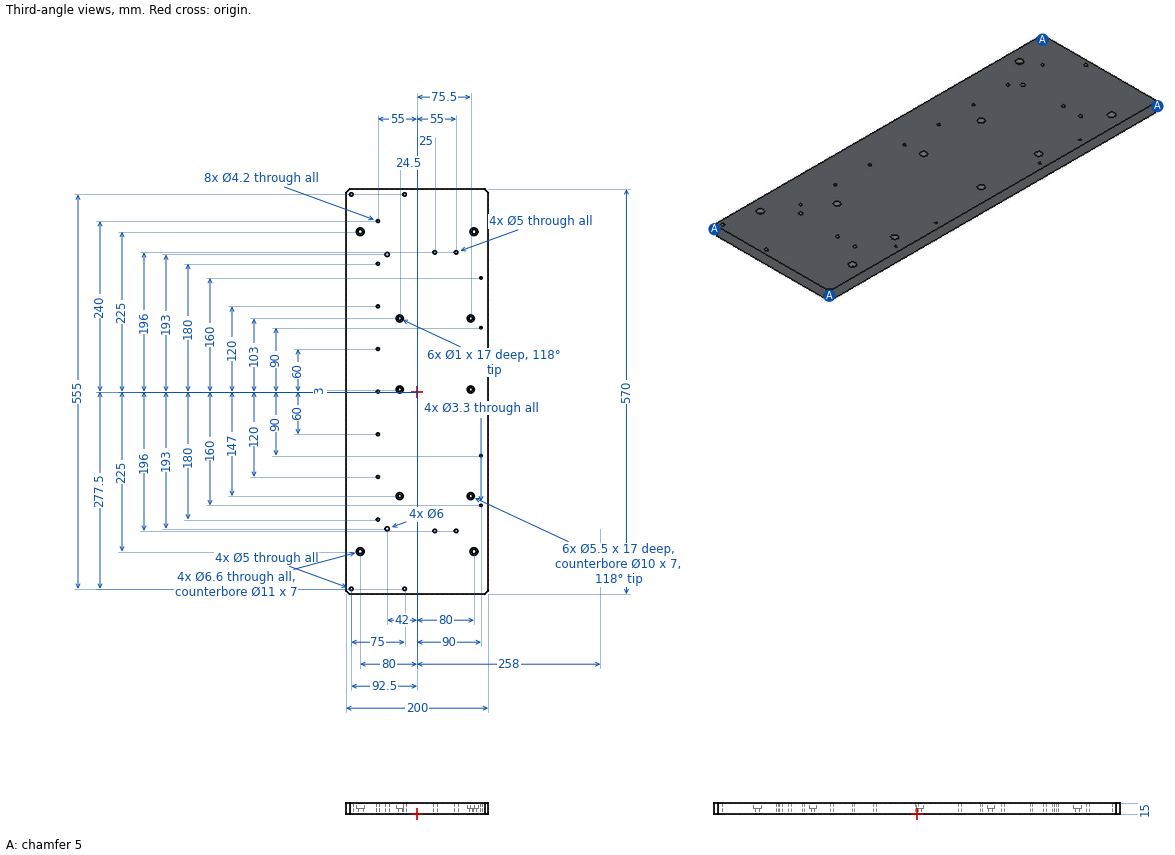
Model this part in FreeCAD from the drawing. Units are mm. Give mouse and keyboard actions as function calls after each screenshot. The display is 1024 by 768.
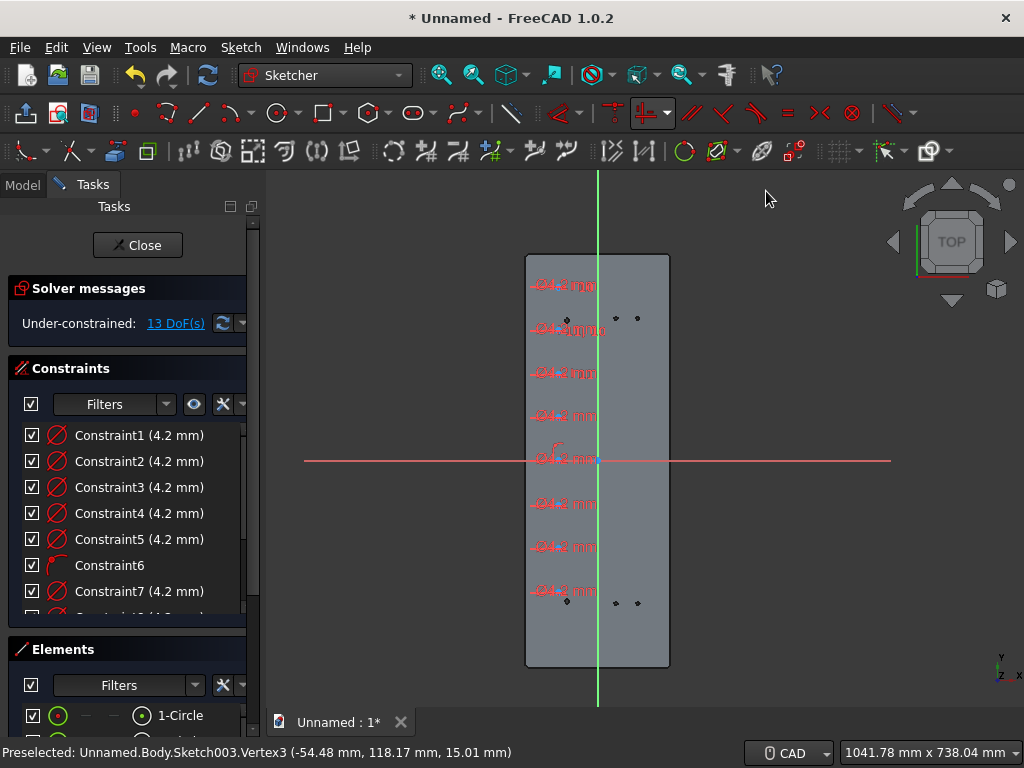
click(558, 375)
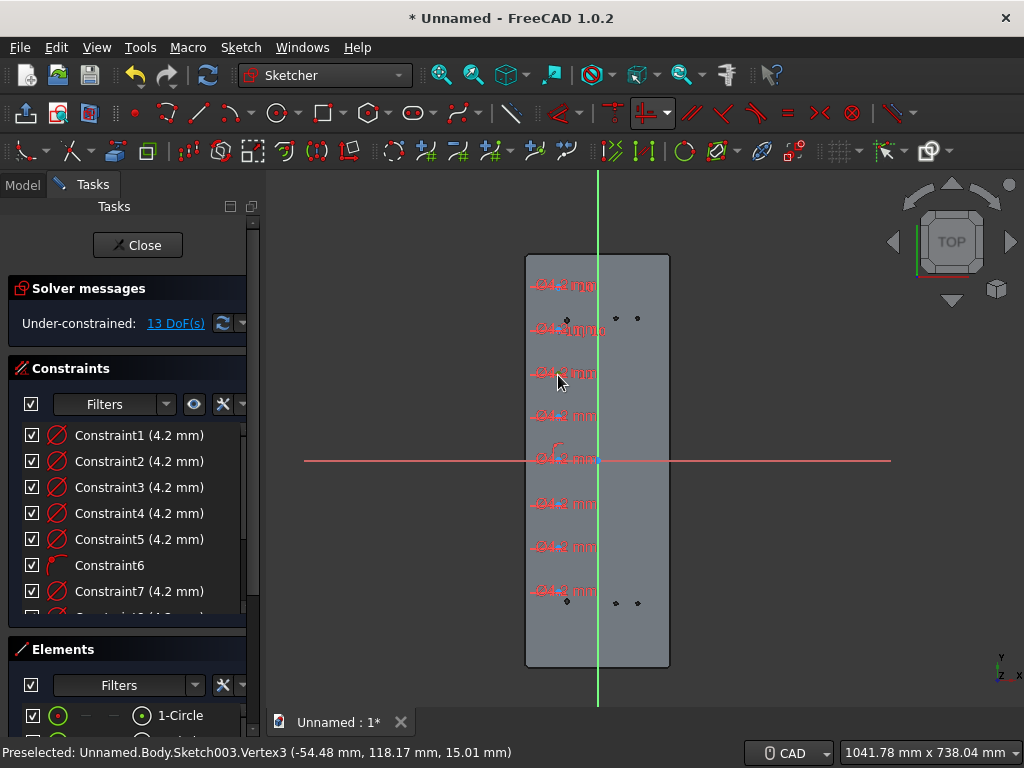
click(558, 418)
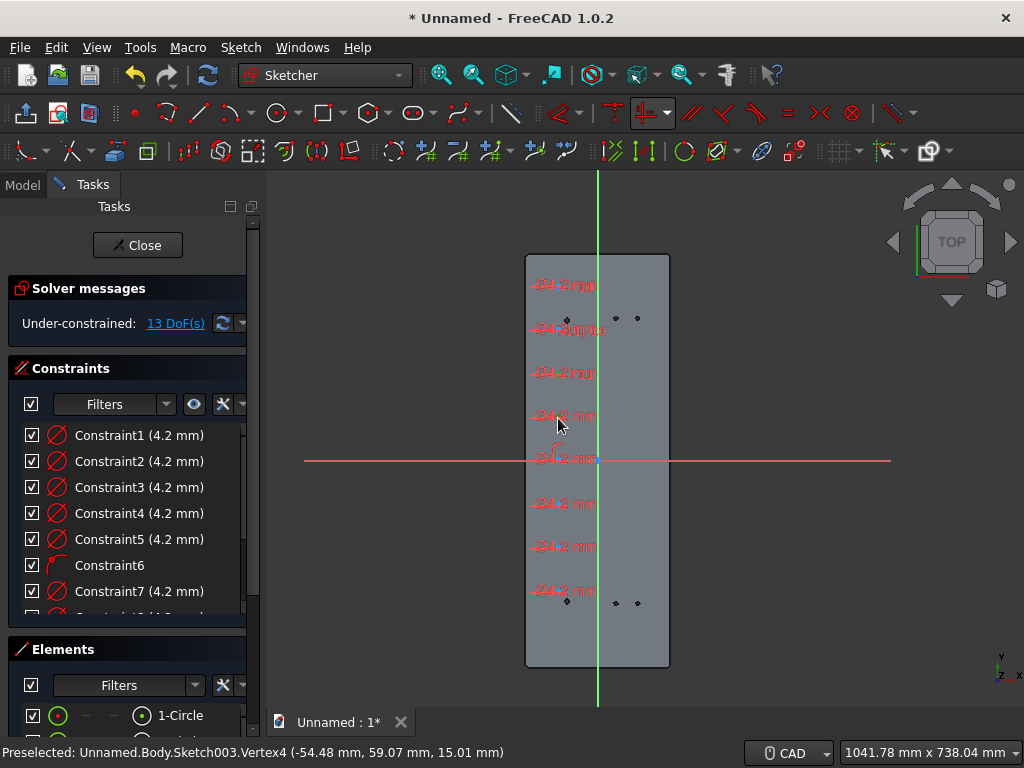
key(v)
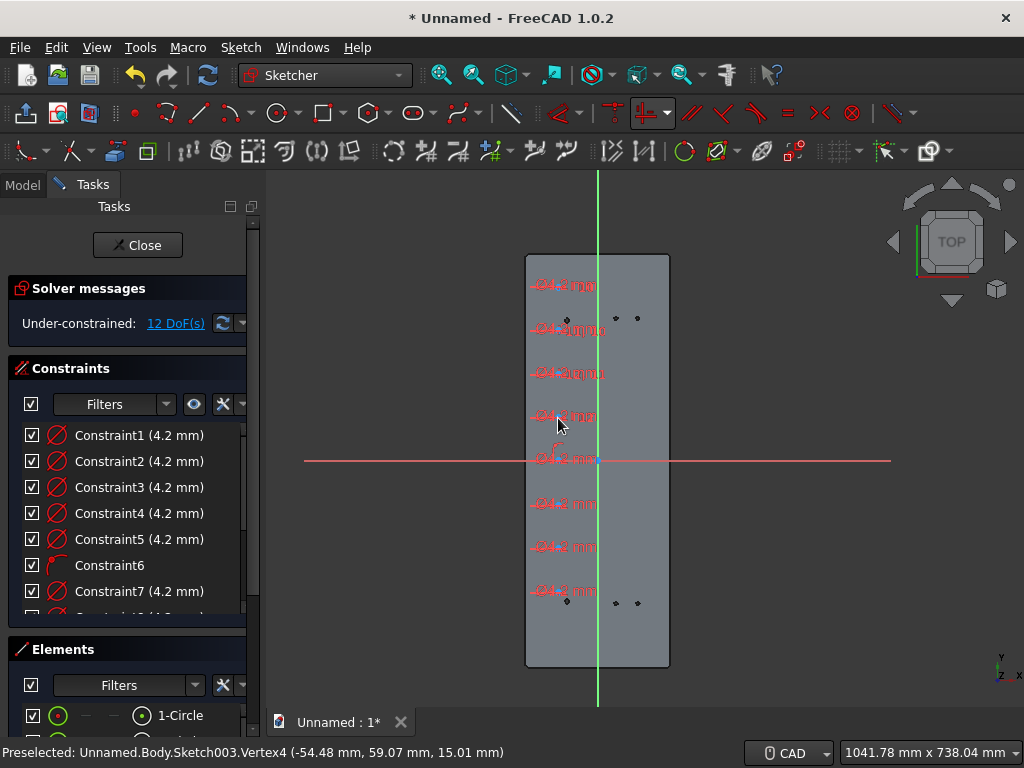
click(558, 418)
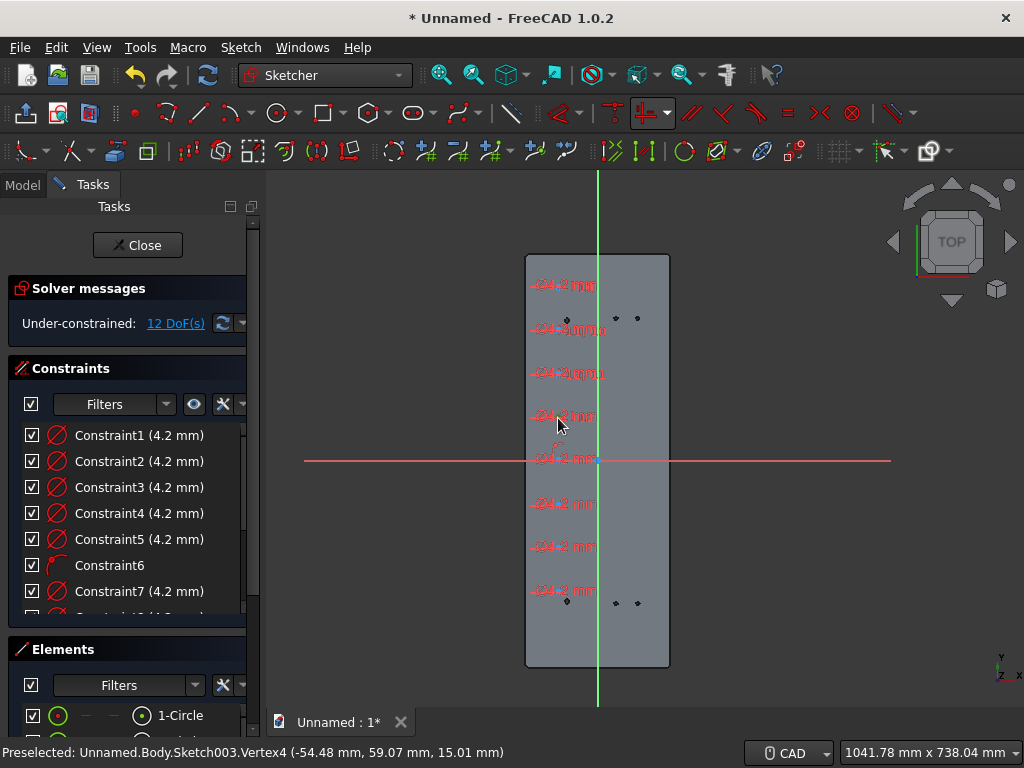
click(558, 461)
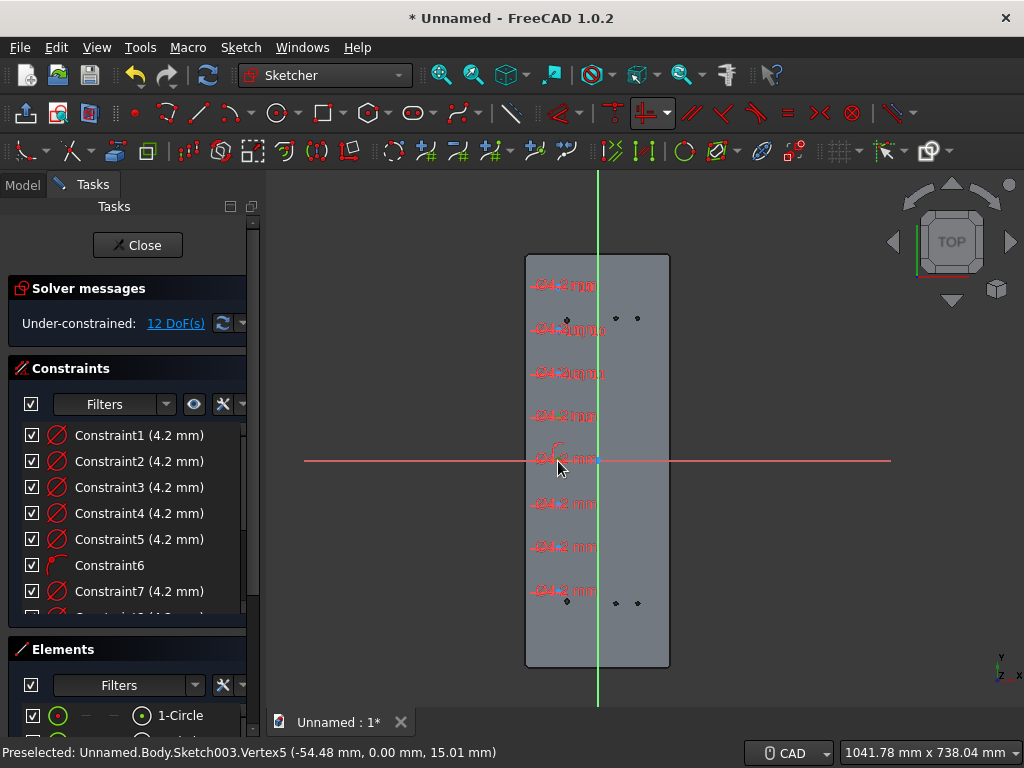
key(v)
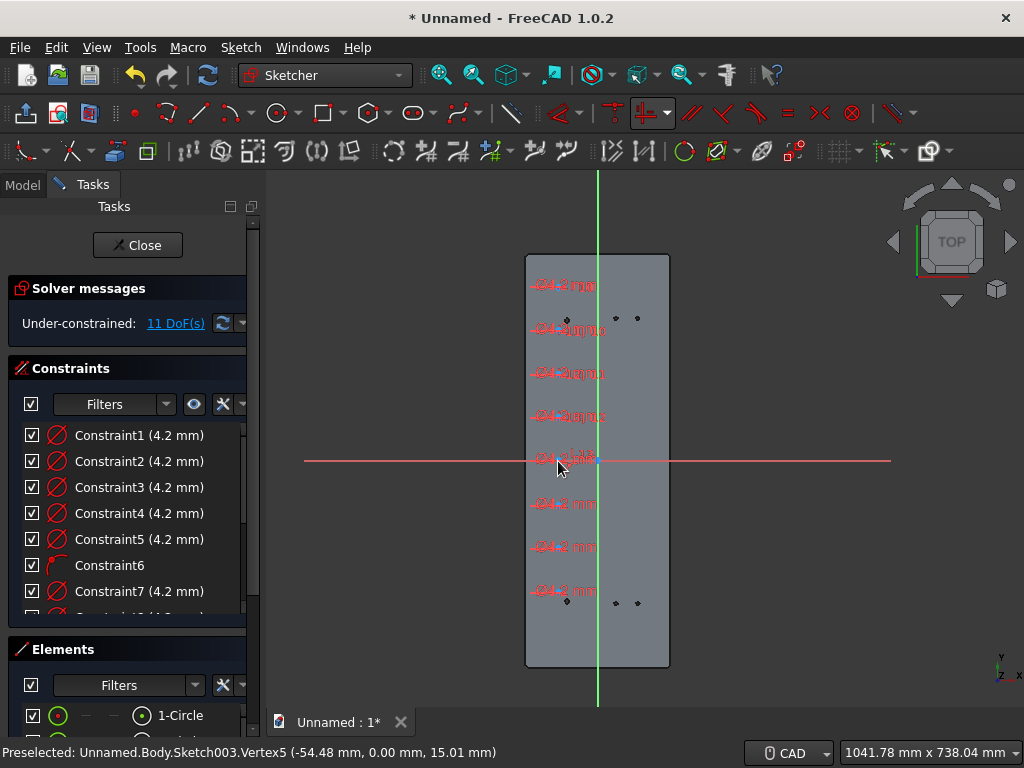
click(558, 461)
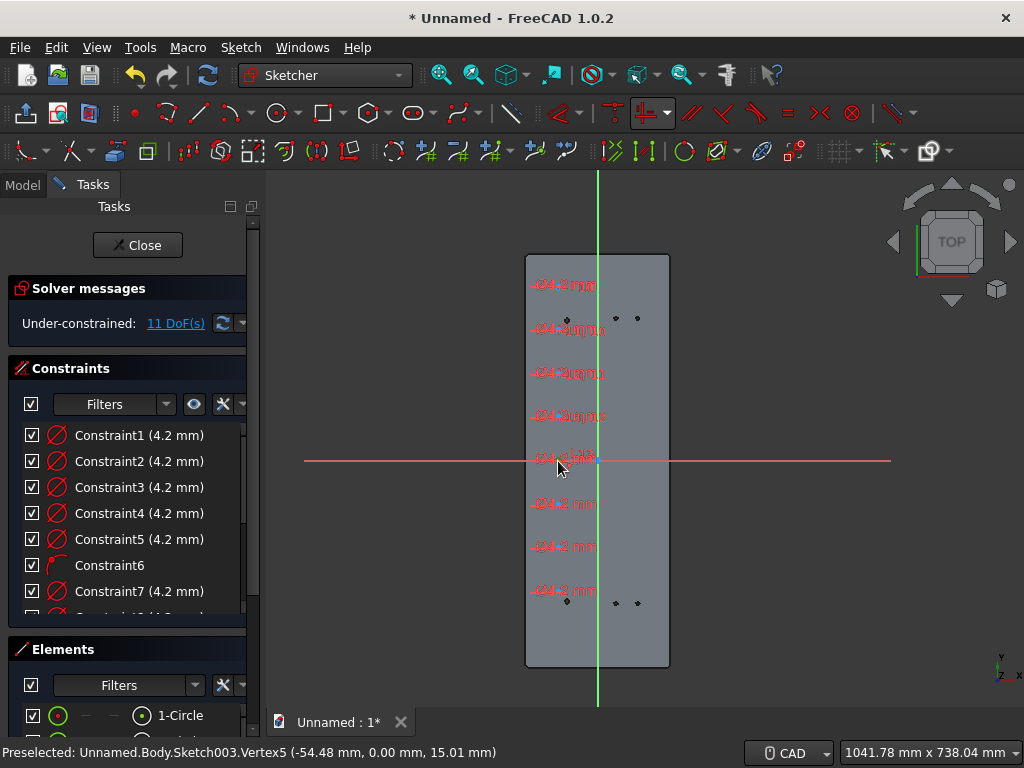
click(558, 506)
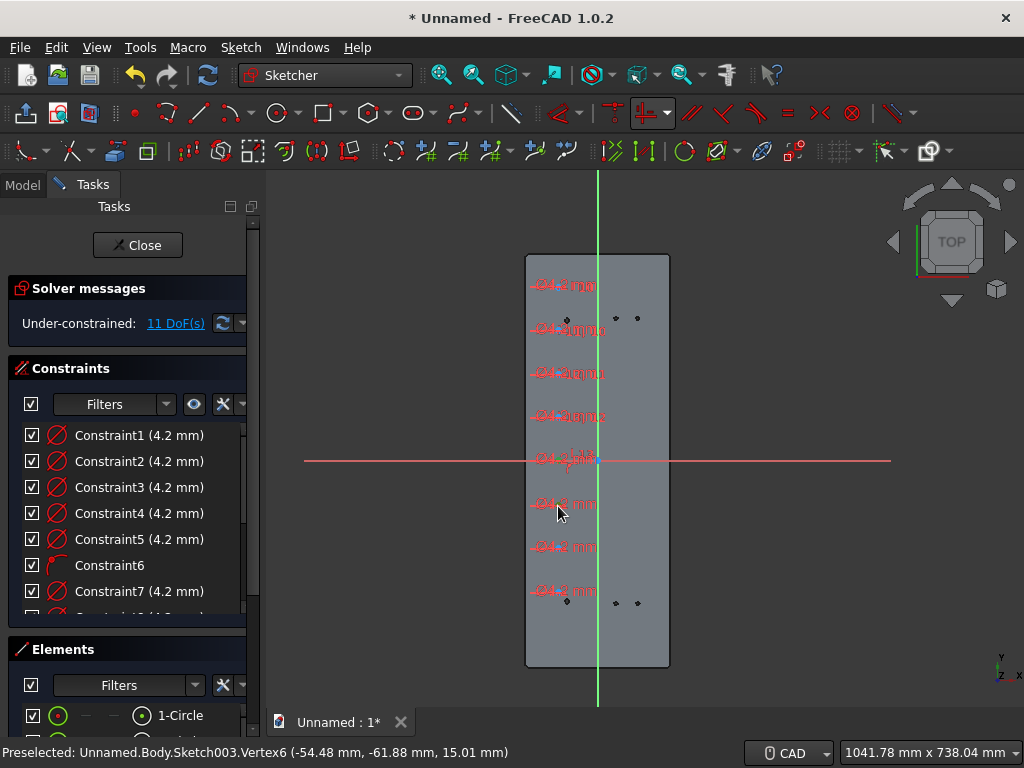
click(670, 114)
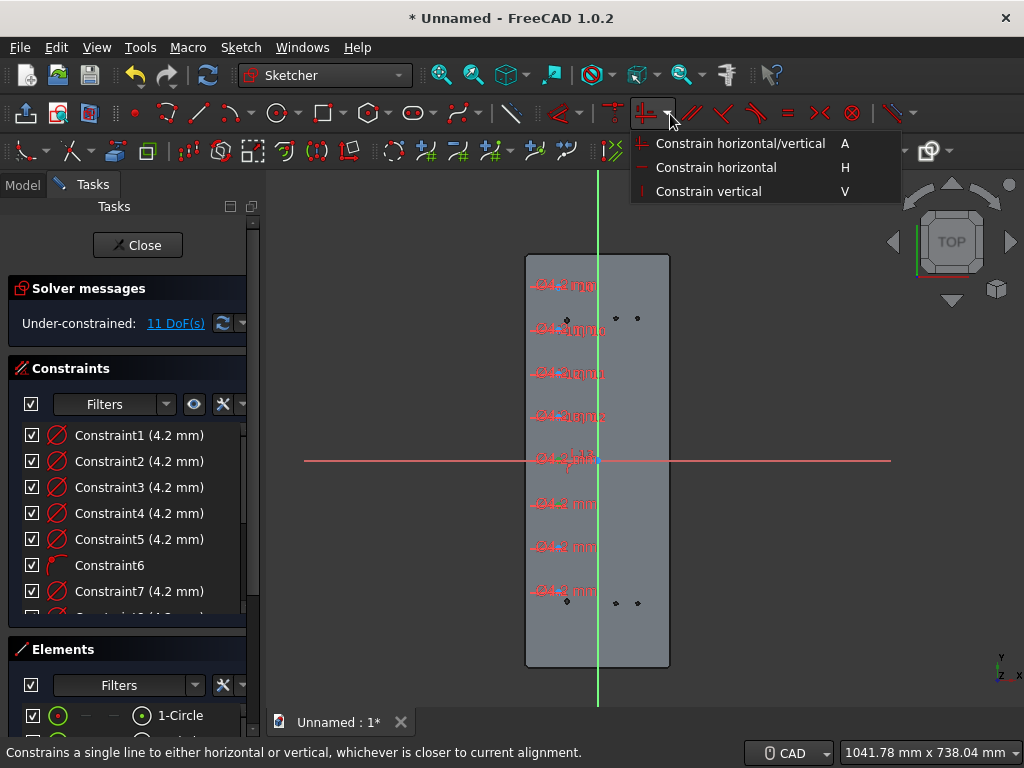
click(766, 191)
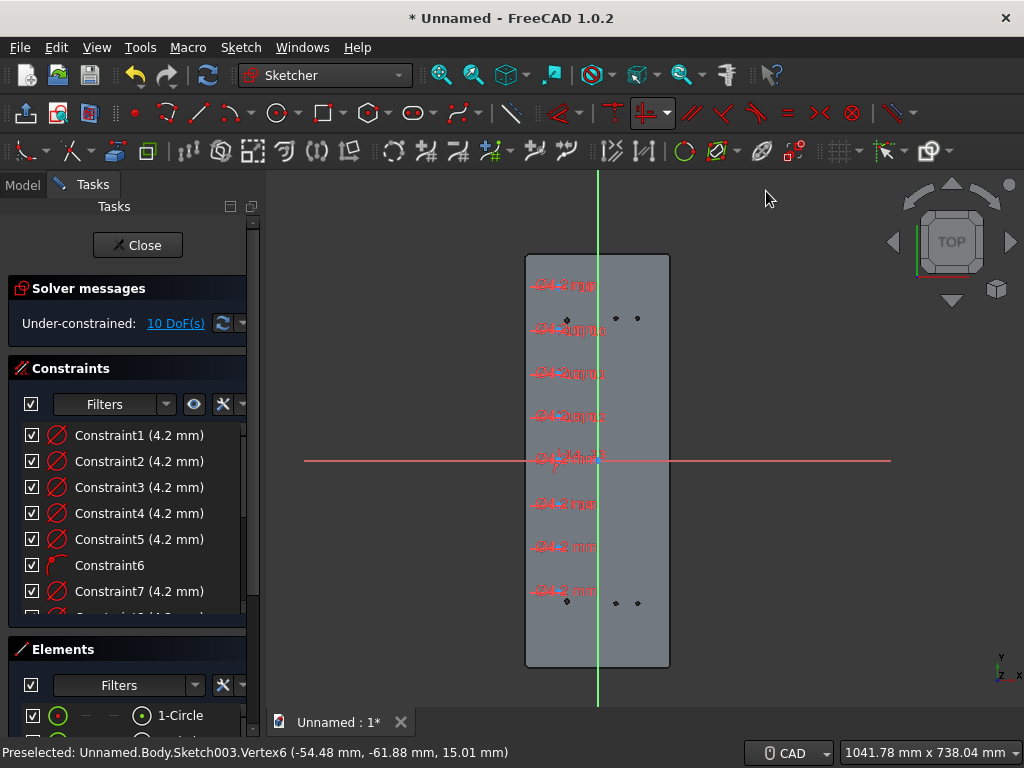
click(558, 506)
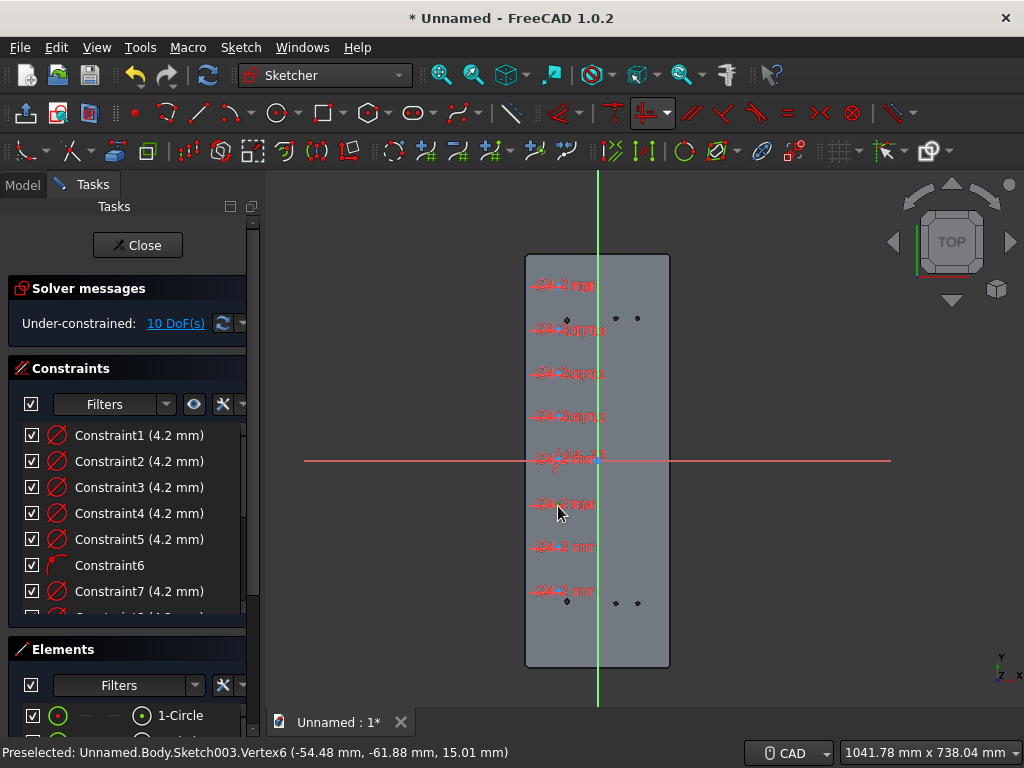
click(558, 549)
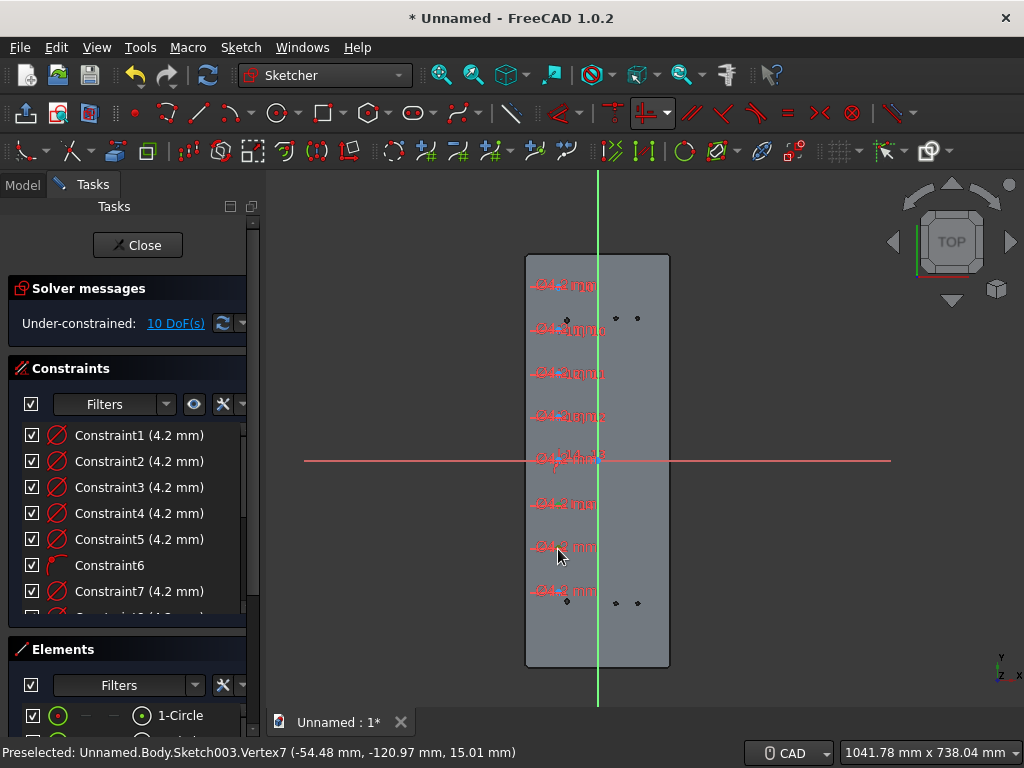
click(670, 114)